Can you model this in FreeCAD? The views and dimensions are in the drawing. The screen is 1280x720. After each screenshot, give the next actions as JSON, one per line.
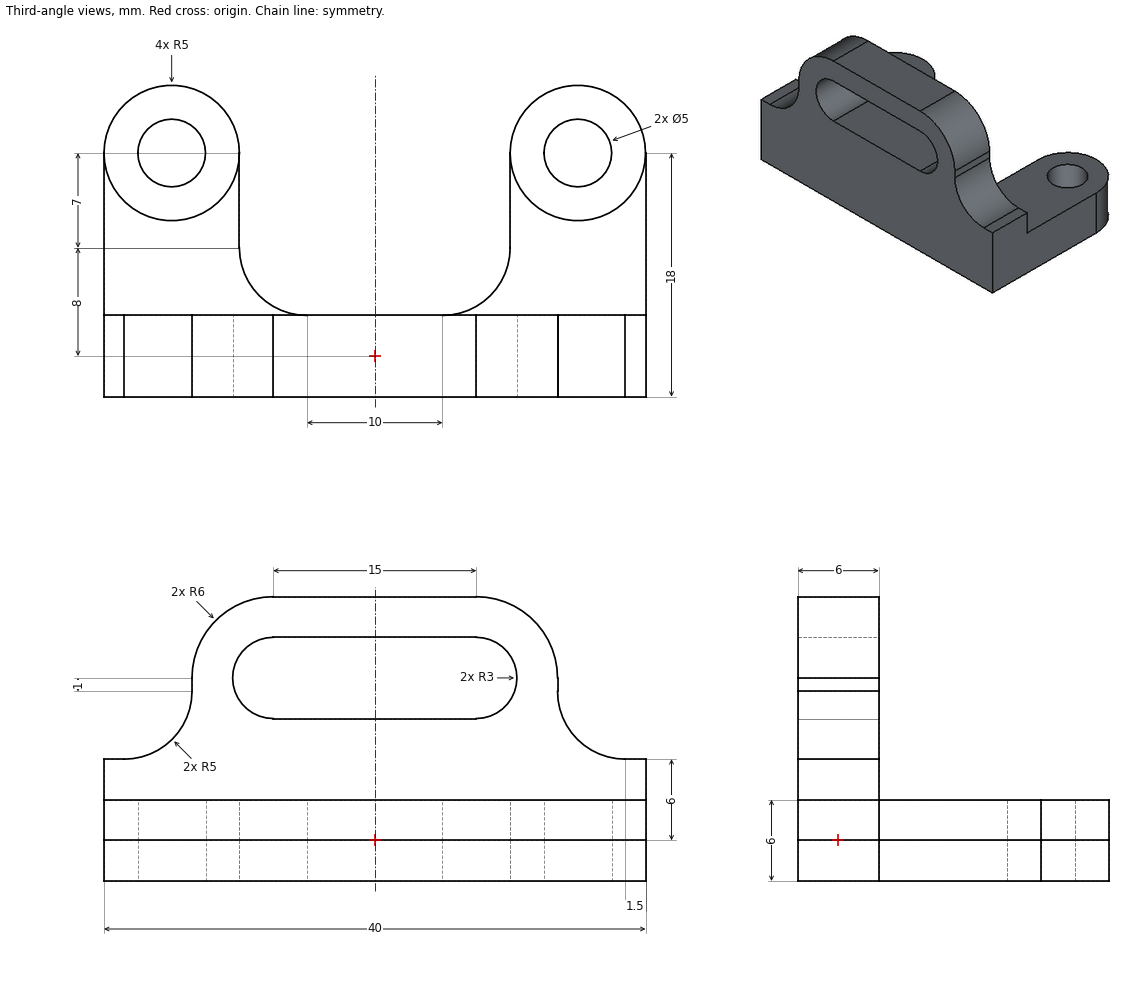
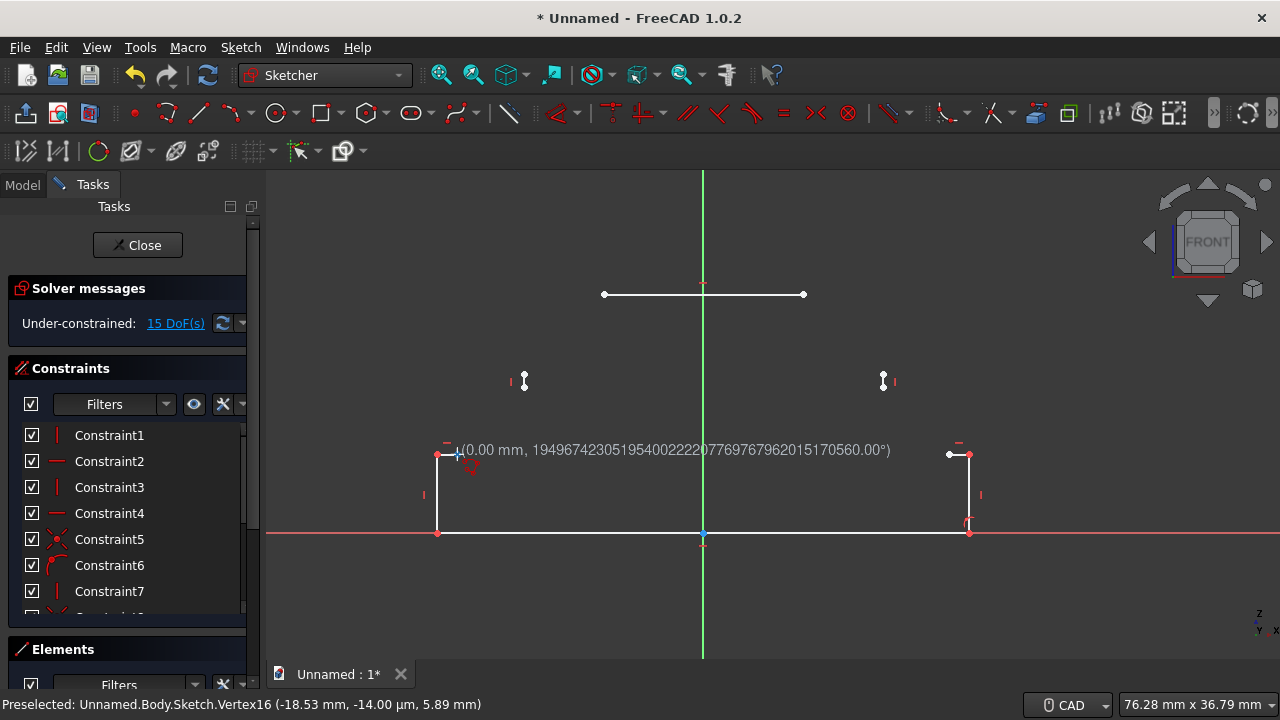
{"action": "left_click", "coordinate": [232, 114]}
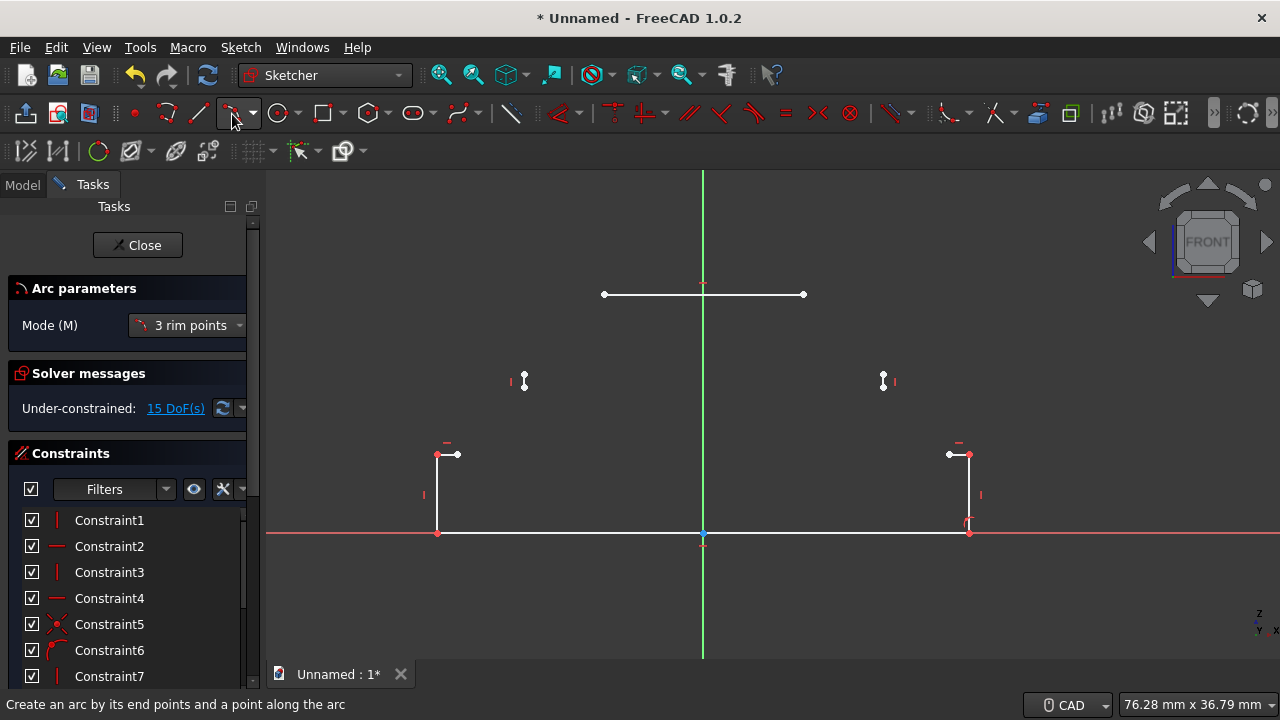
{"action": "scroll", "coordinate": [524, 374], "scroll_direction": "up", "scroll_amount": 5}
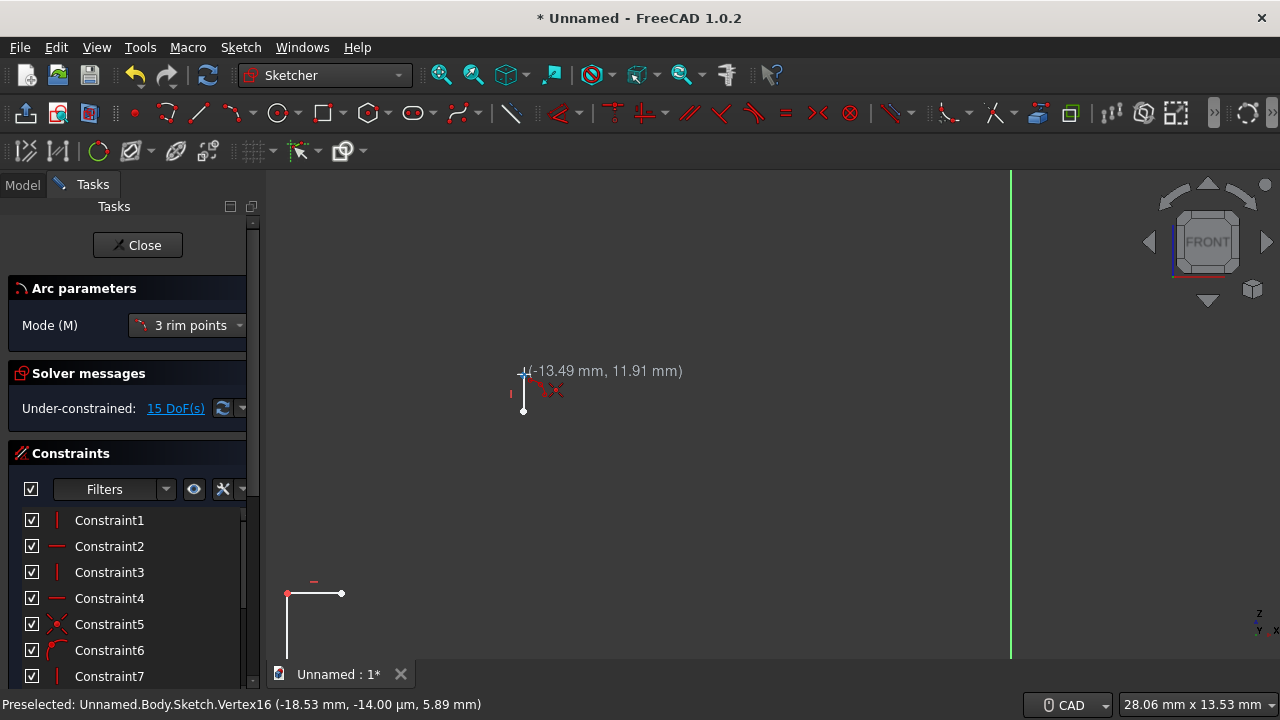
{"action": "left_click", "coordinate": [524, 376]}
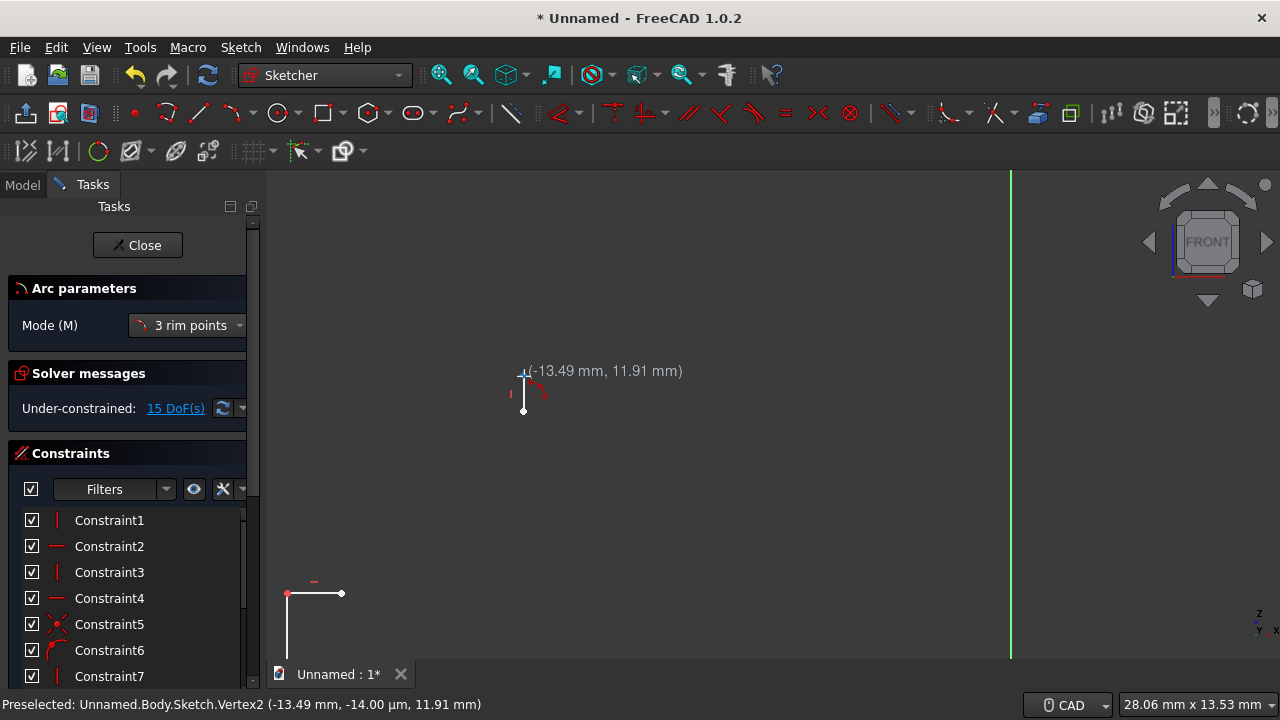
{"action": "scroll", "coordinate": [526, 376], "scroll_direction": "down", "scroll_amount": 5}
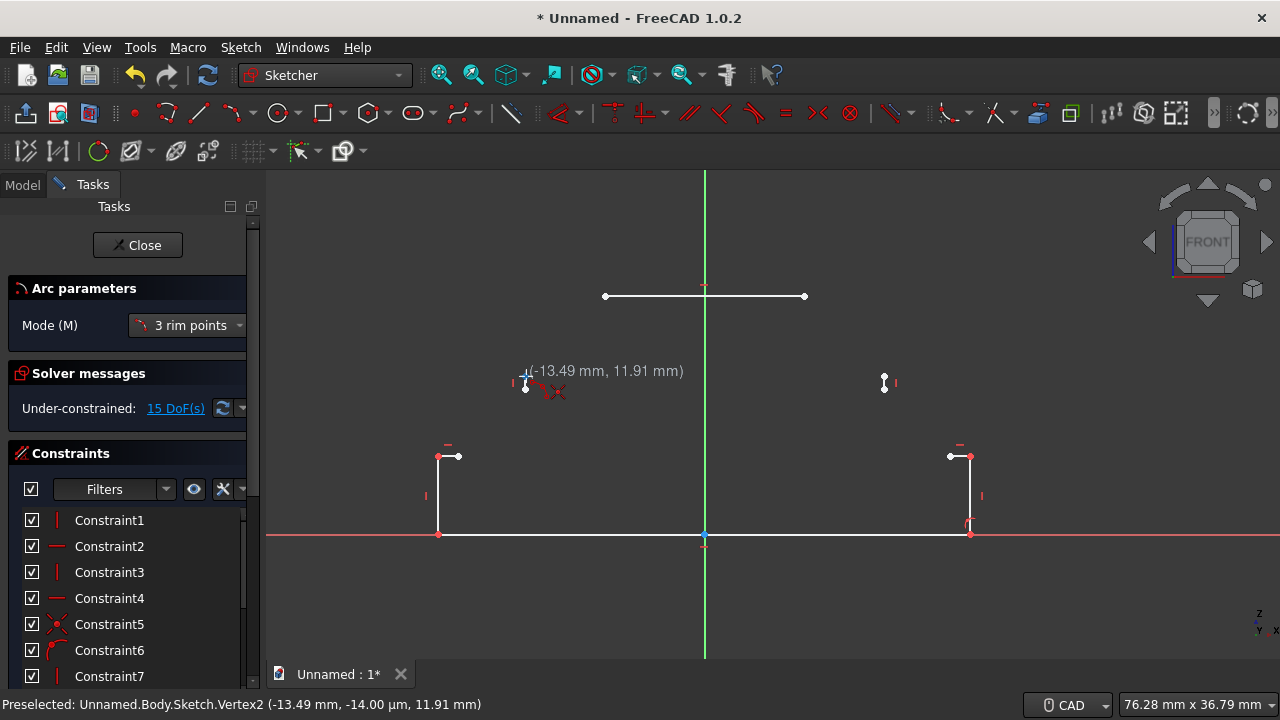
{"action": "left_click", "coordinate": [605, 296]}
{"action": "left_click", "coordinate": [549, 319]}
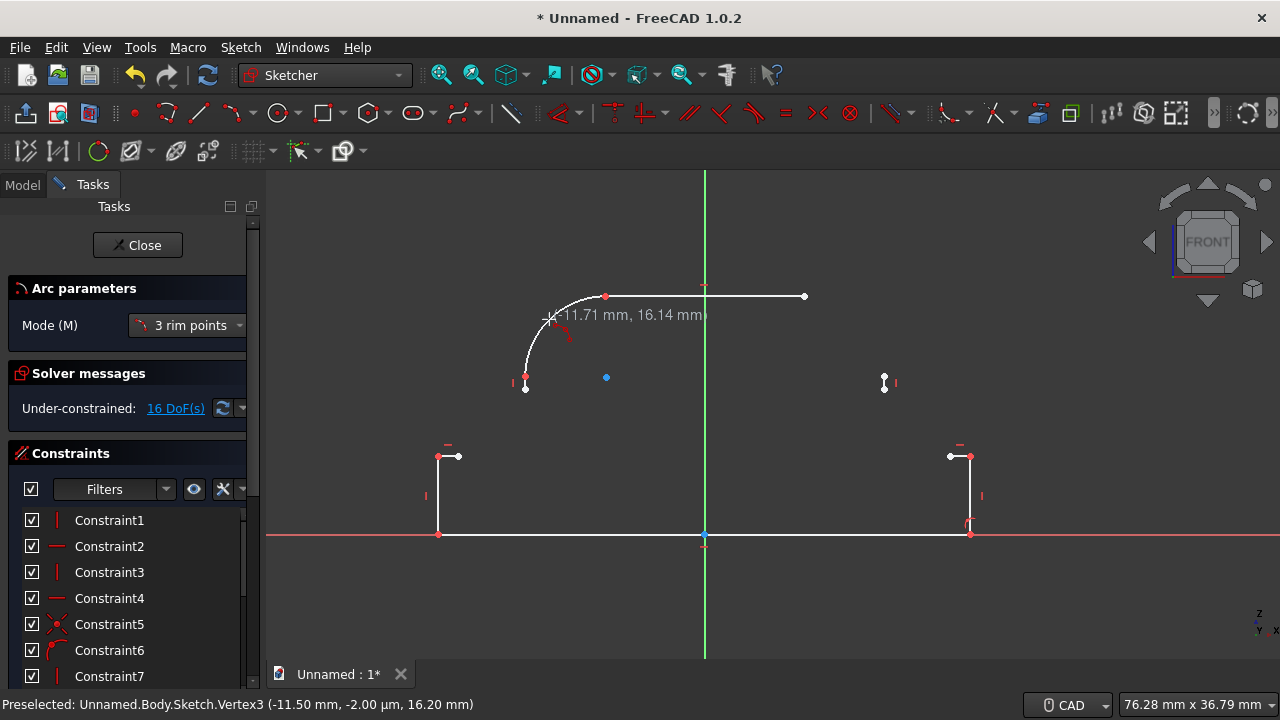
{"action": "left_click", "coordinate": [804, 296]}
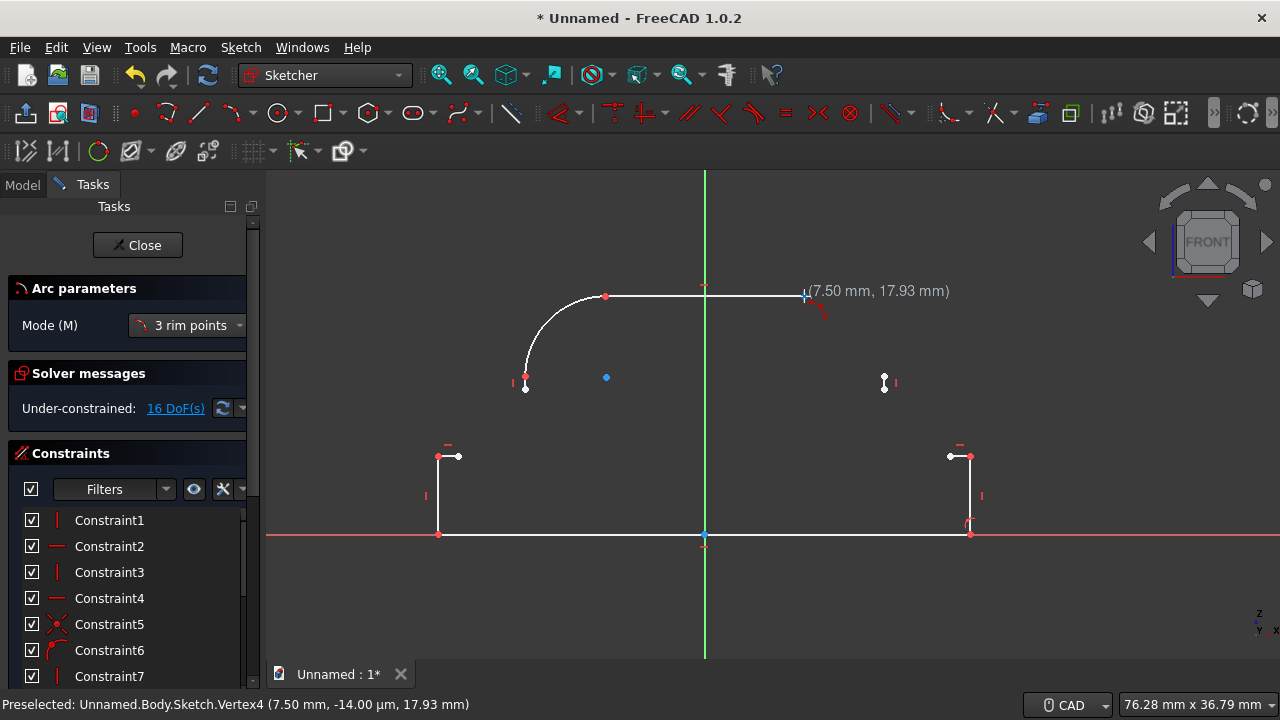
{"action": "scroll", "coordinate": [884, 375], "scroll_direction": "up", "scroll_amount": 5}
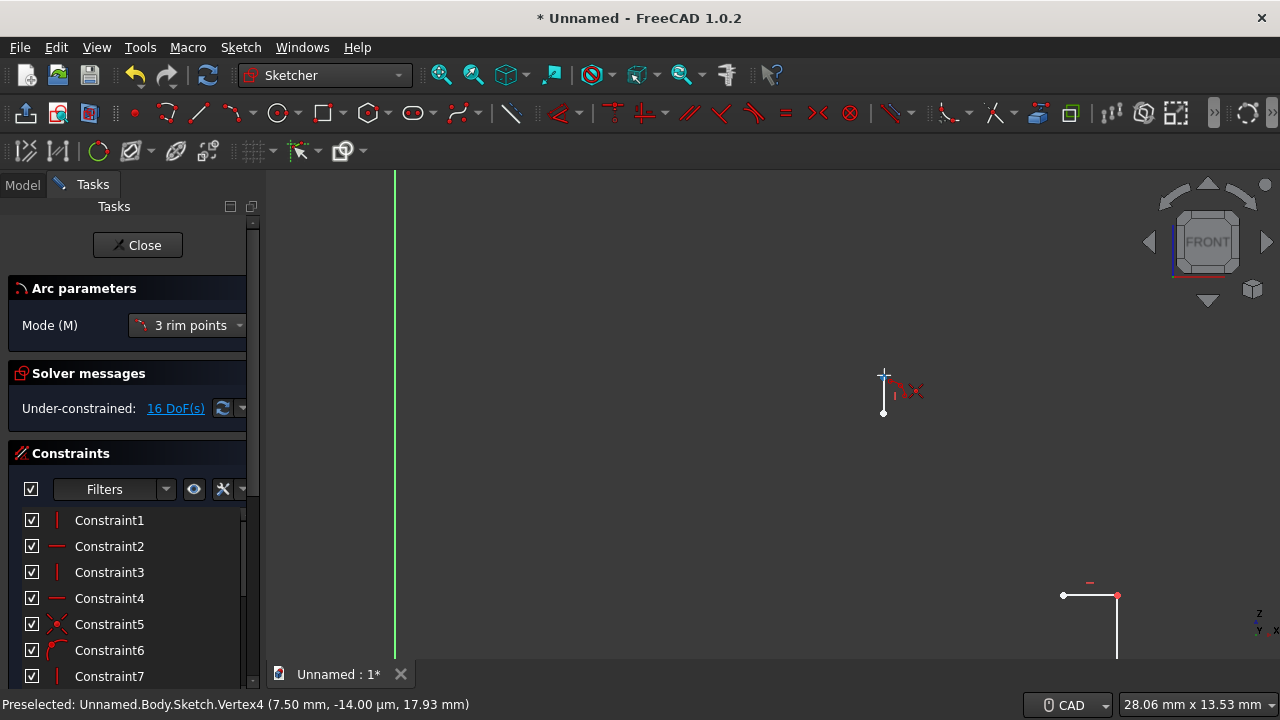
{"action": "left_click", "coordinate": [884, 378]}
{"action": "left_click", "coordinate": [820, 221]}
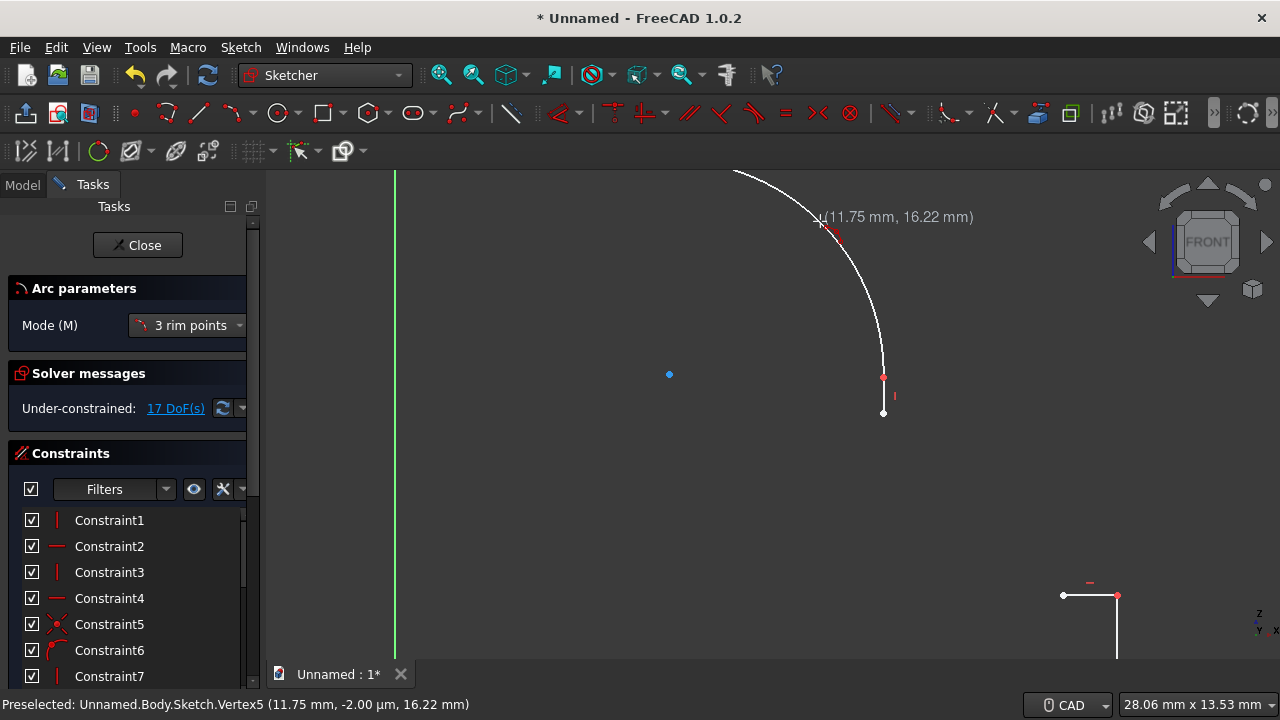
{"action": "left_click", "coordinate": [884, 413]}
{"action": "left_click", "coordinate": [1063, 595]}
{"action": "left_click", "coordinate": [936, 538]}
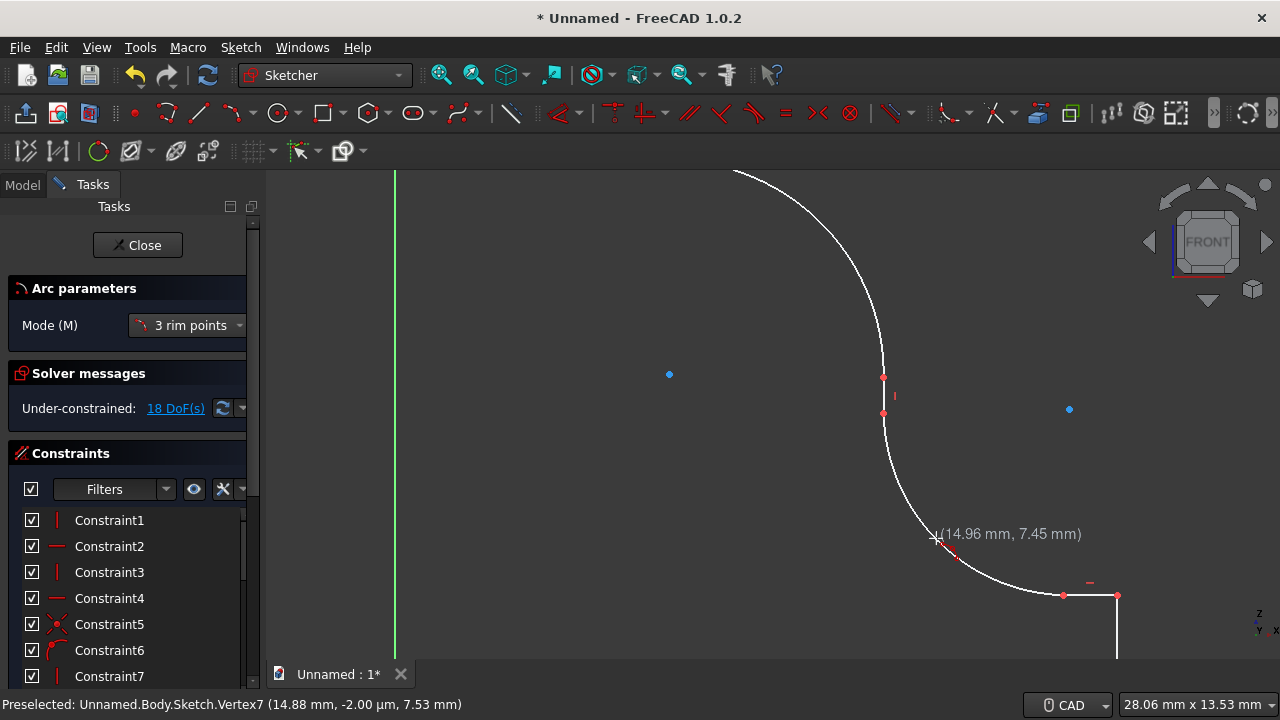
{"action": "scroll", "coordinate": [884, 375], "scroll_direction": "down", "scroll_amount": 5}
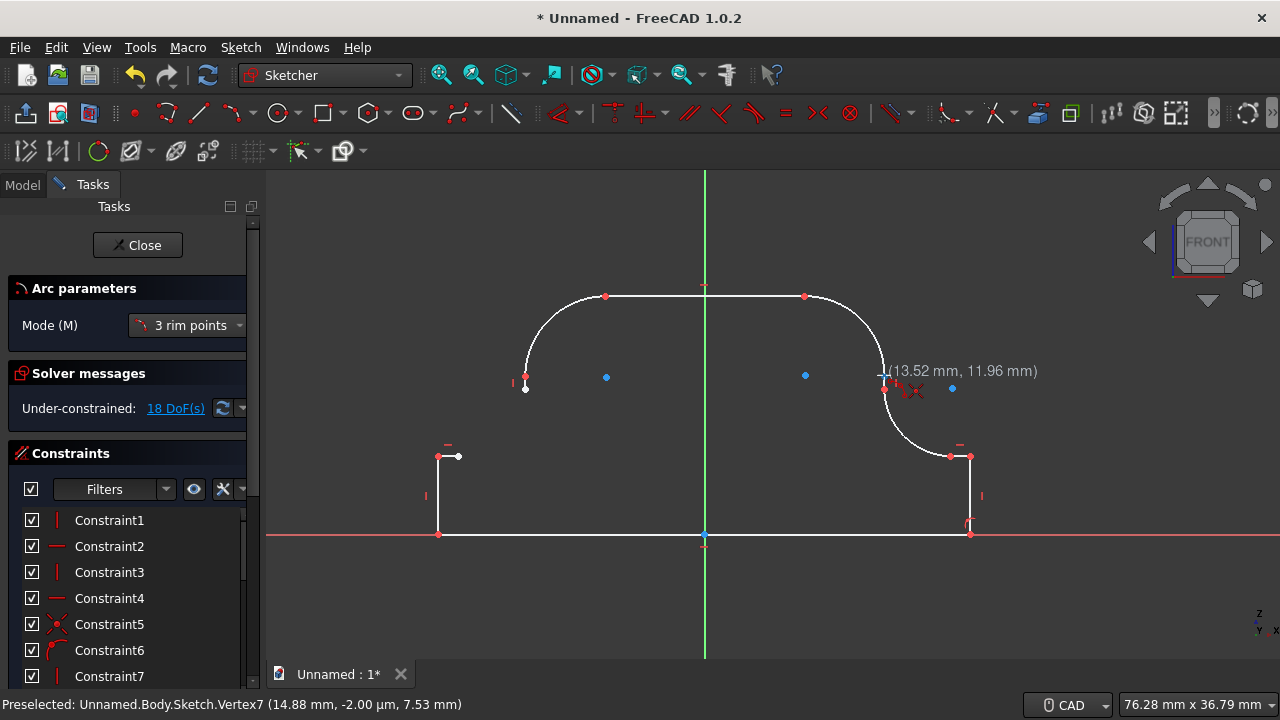
{"action": "scroll", "coordinate": [459, 455], "scroll_direction": "up", "scroll_amount": 3}